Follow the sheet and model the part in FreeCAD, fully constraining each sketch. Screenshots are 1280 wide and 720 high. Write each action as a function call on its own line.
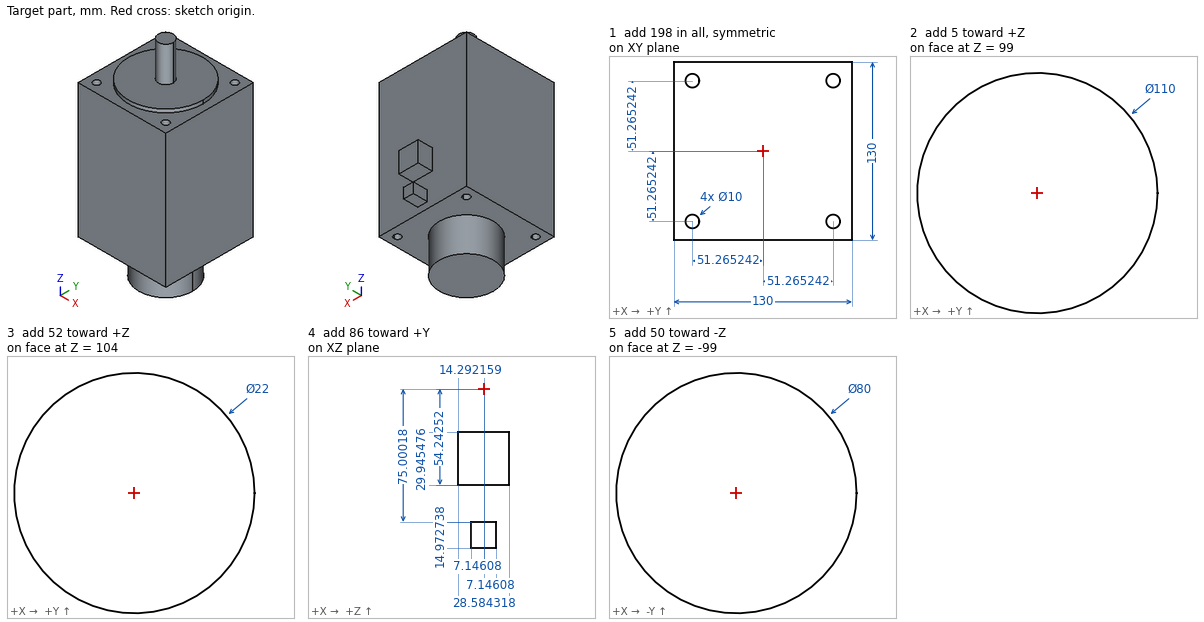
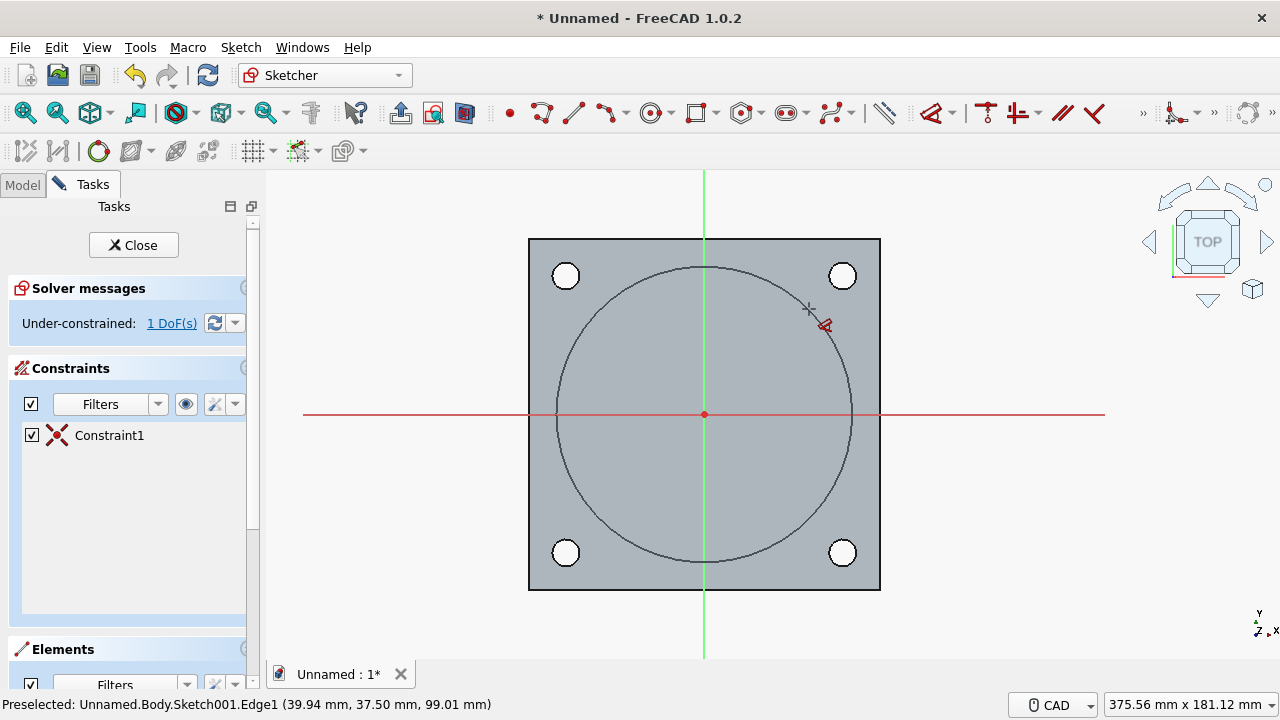
click(809, 310)
click(832, 287)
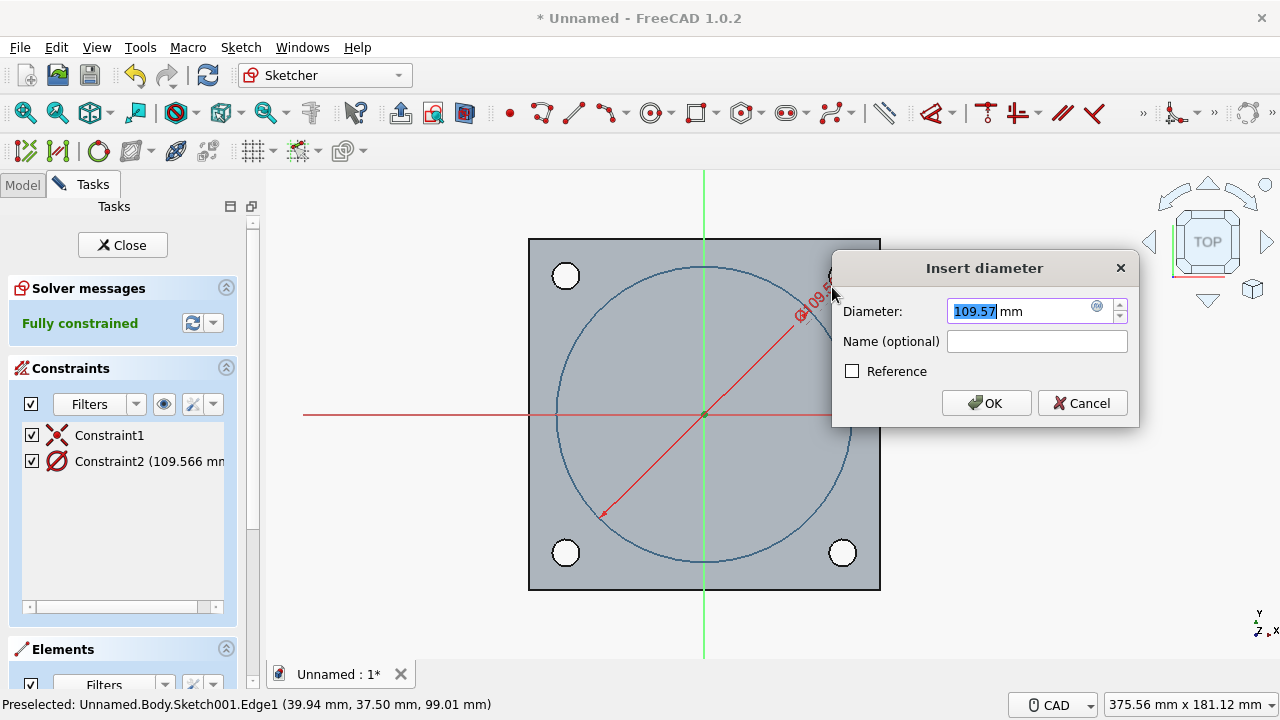
text(110)
key(Return)
key(Escape)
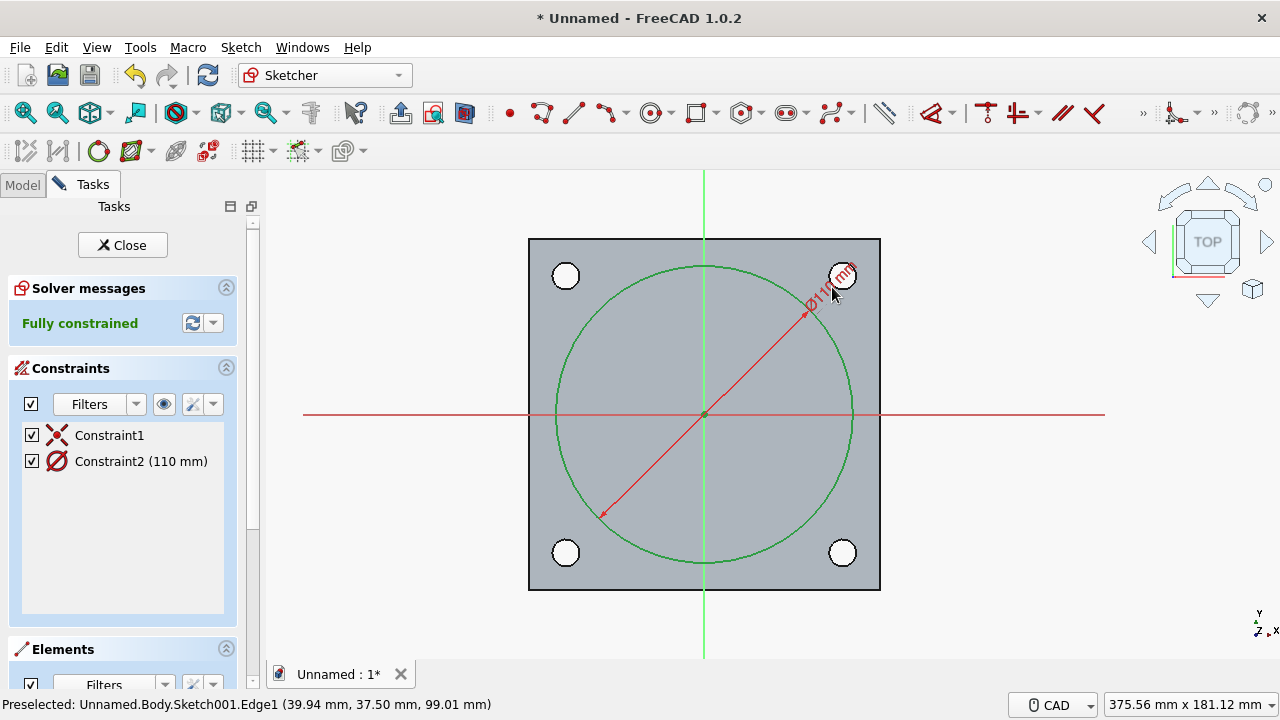
click(123, 245)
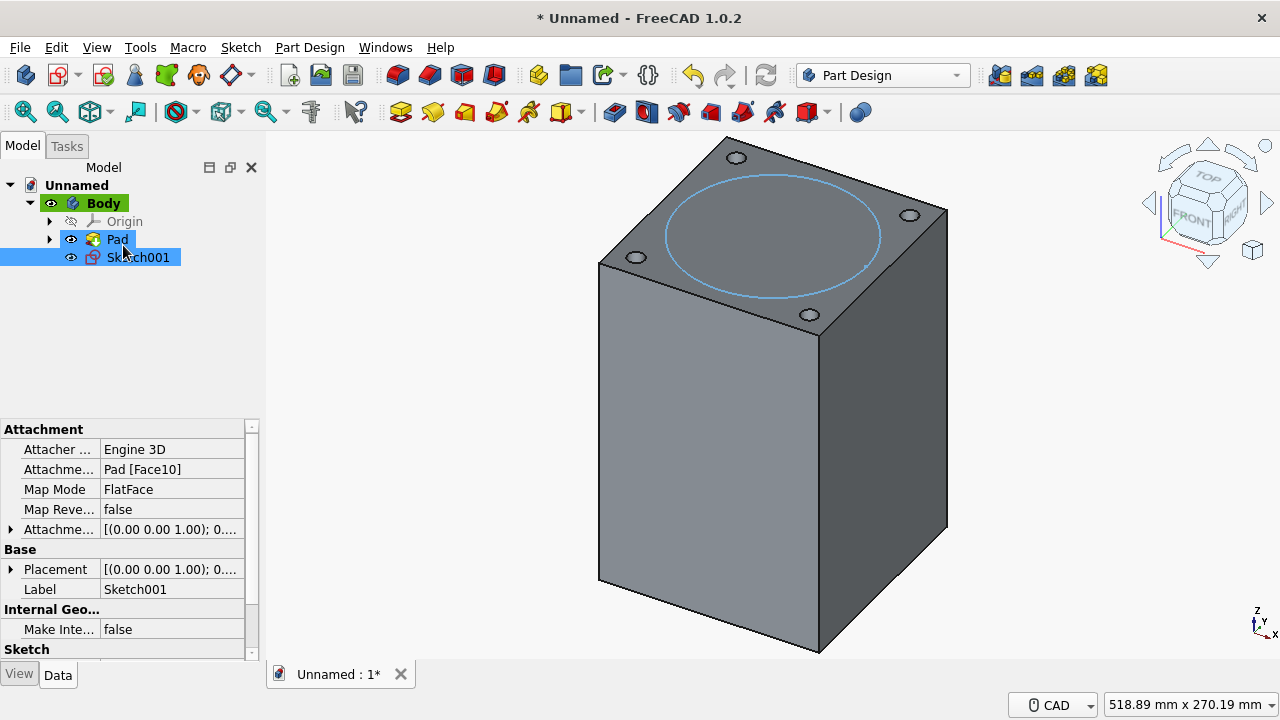
click(402, 112)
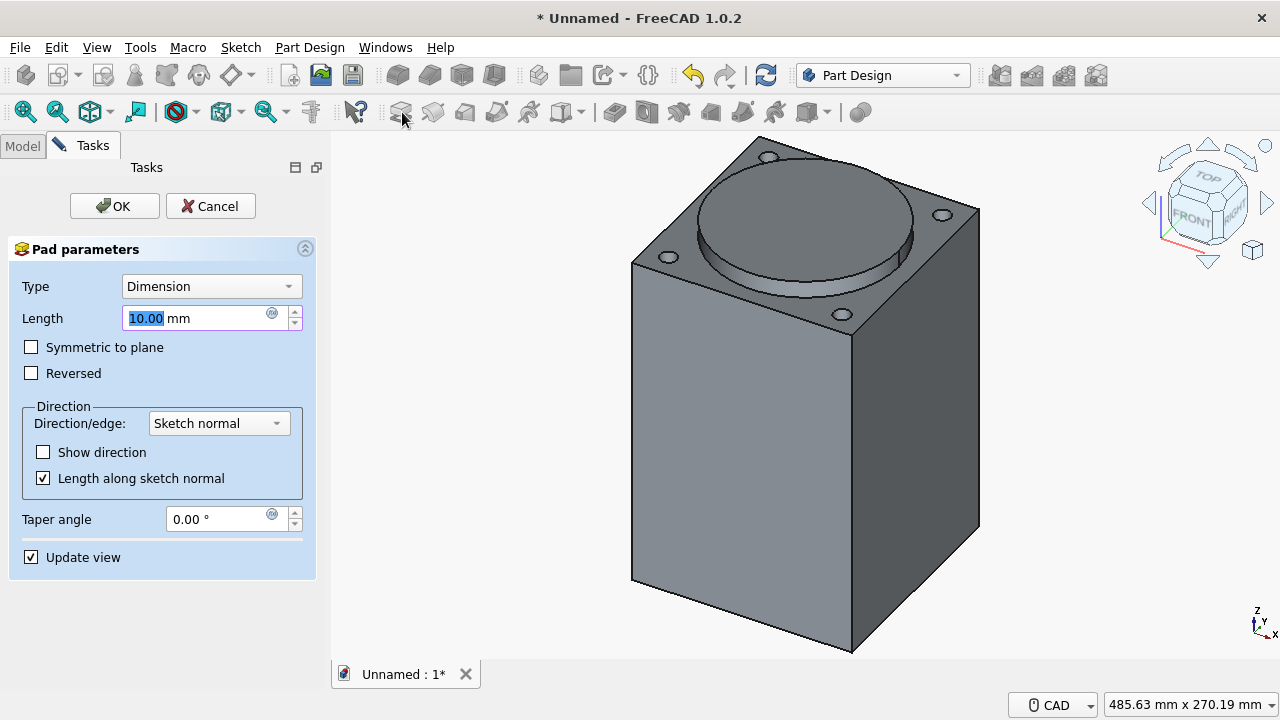
text(5)
key(Tab)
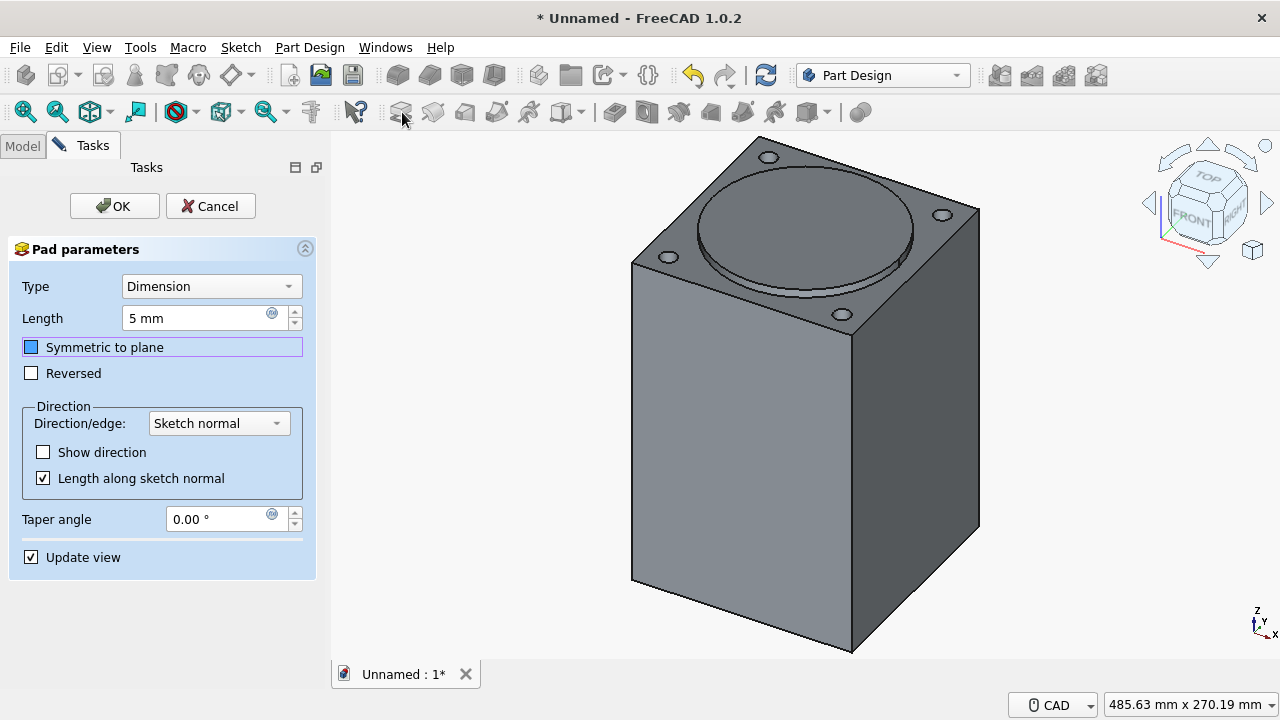
click(115, 206)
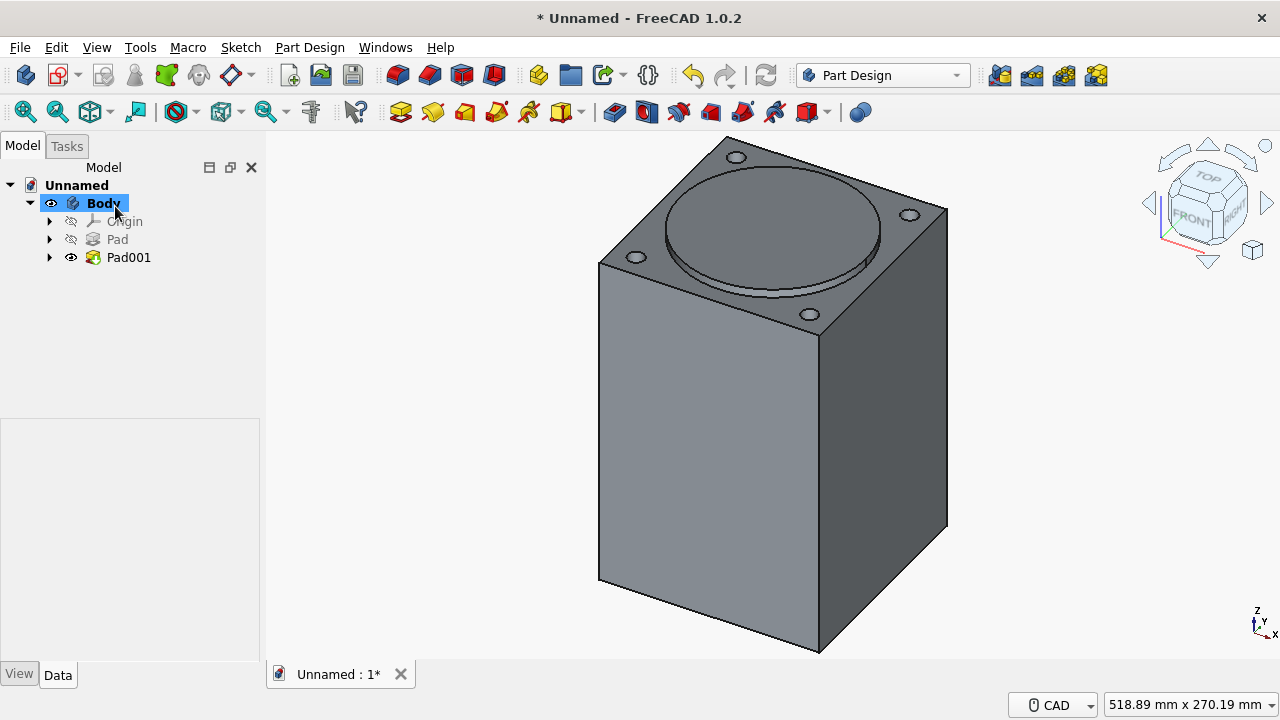
key(v)
key(f)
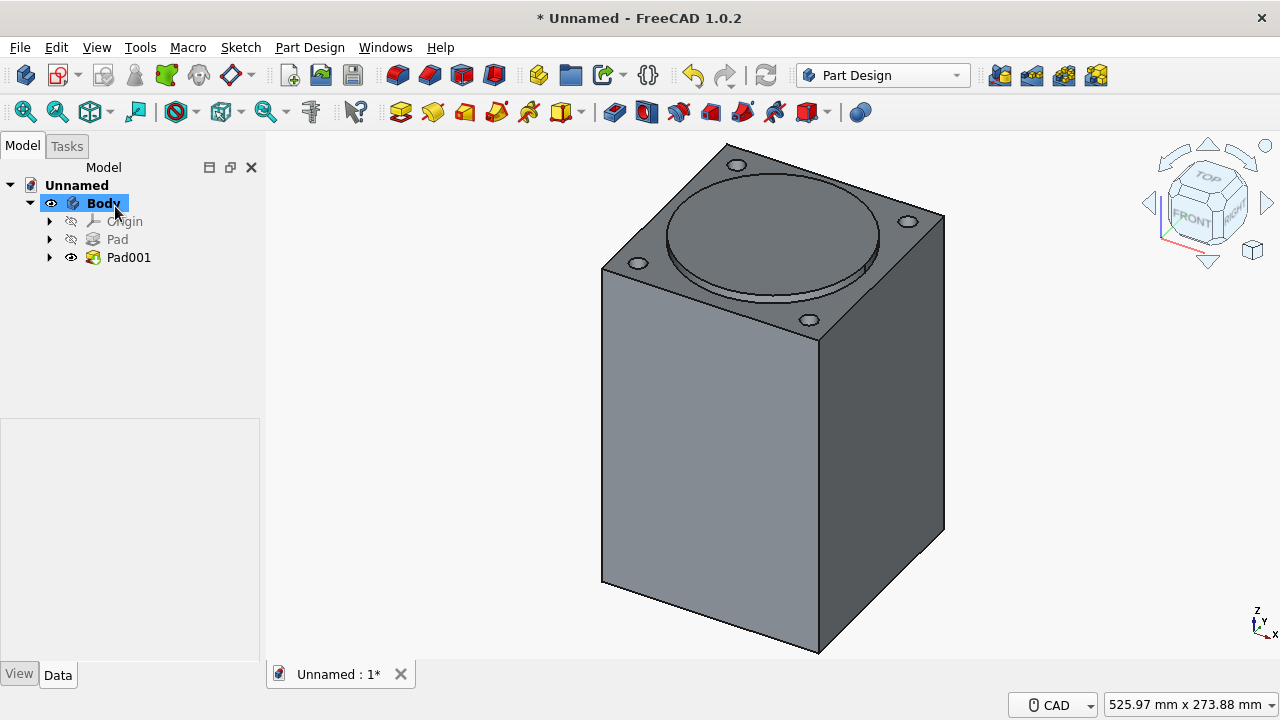
click(773, 234)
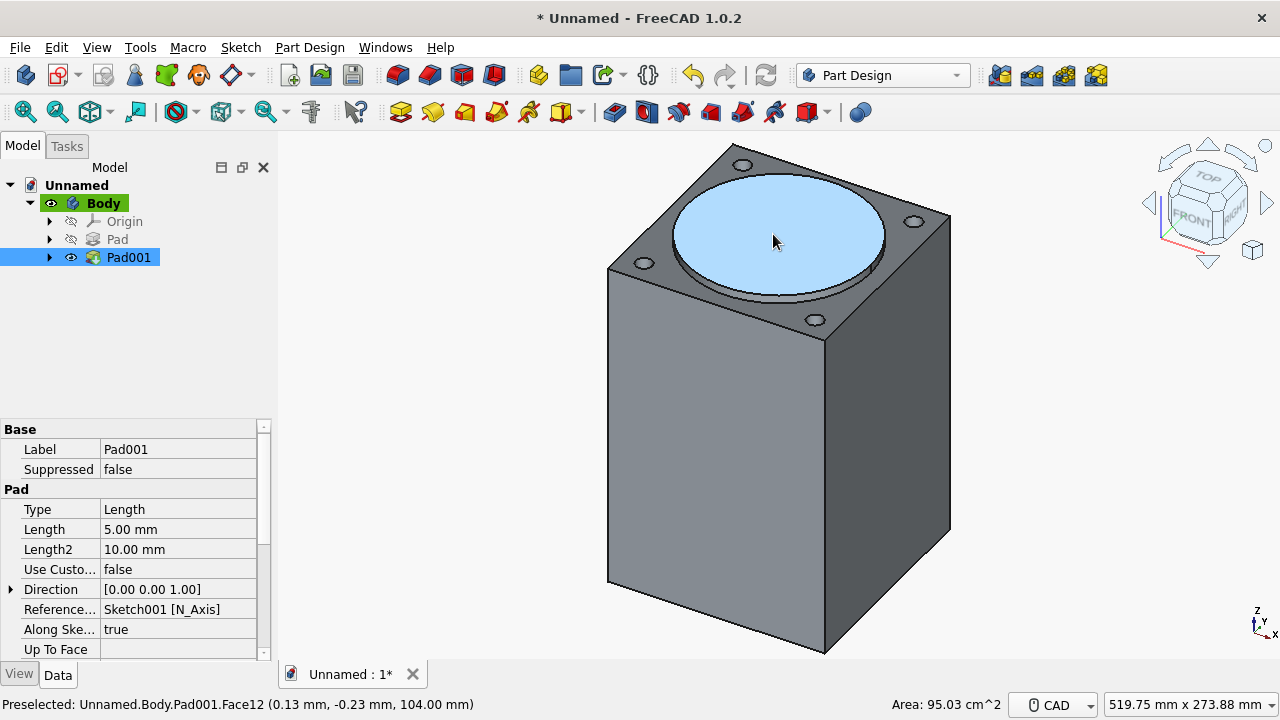
click(58, 76)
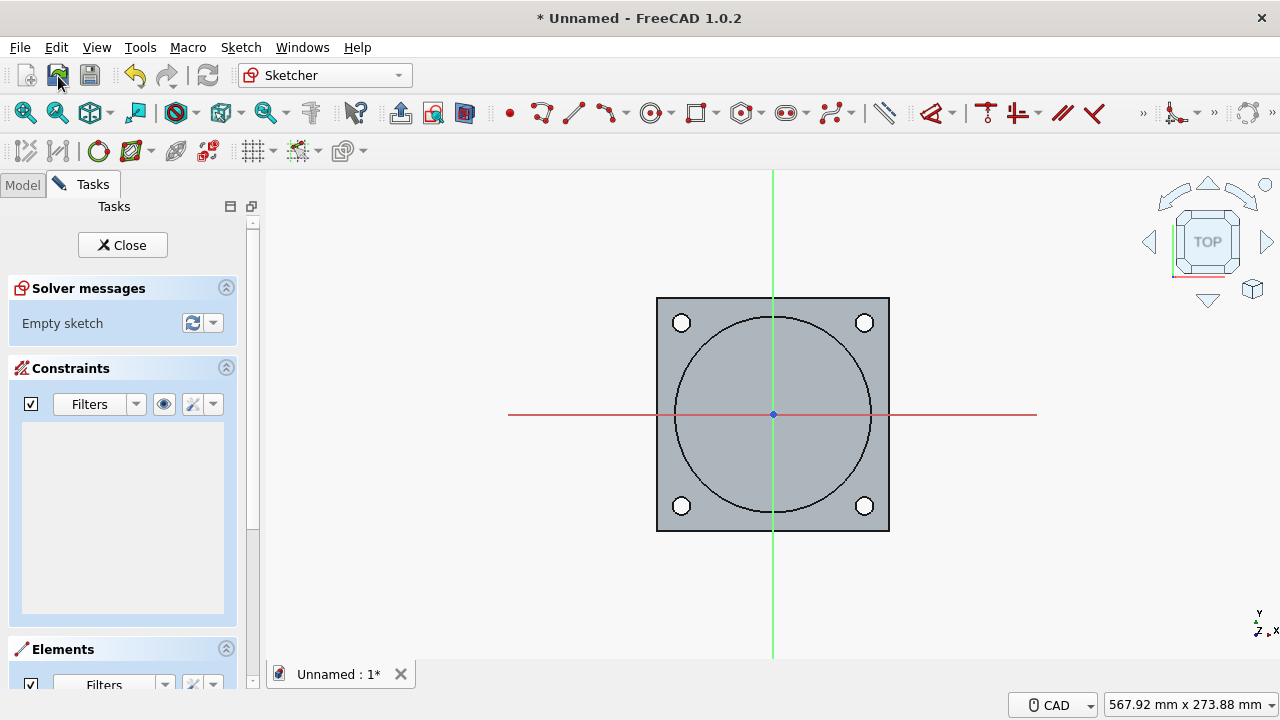
scroll(784, 414, up, 10)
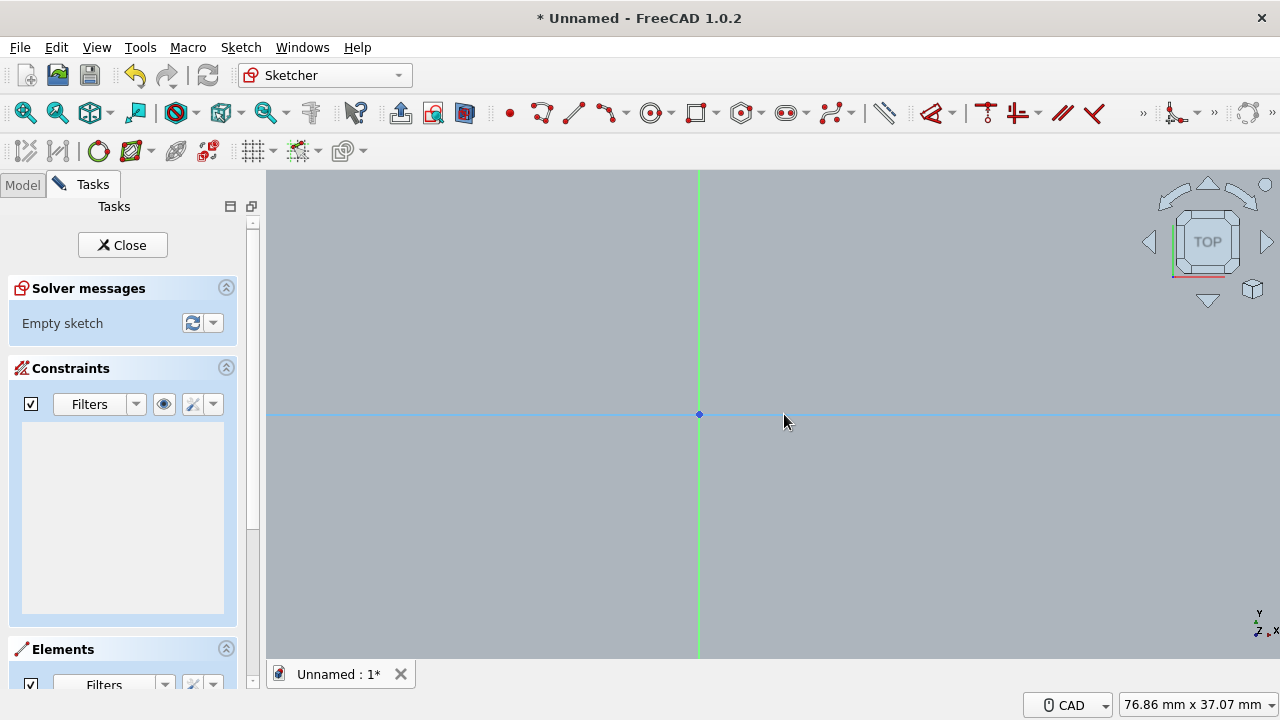
click(652, 114)